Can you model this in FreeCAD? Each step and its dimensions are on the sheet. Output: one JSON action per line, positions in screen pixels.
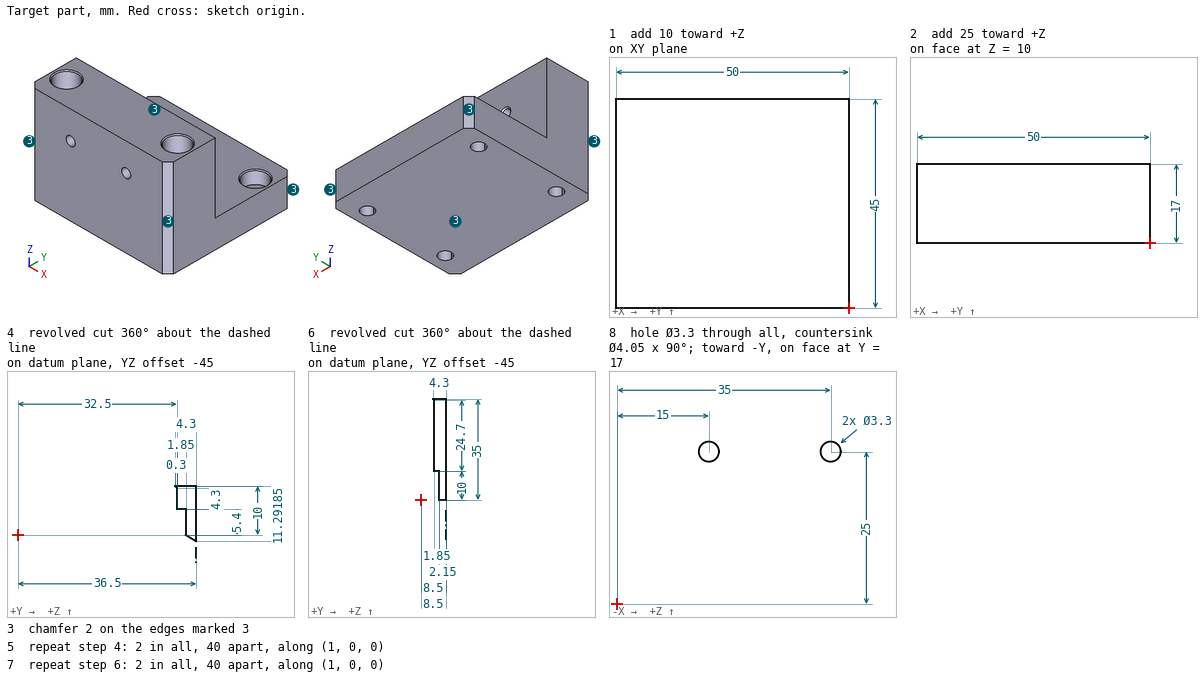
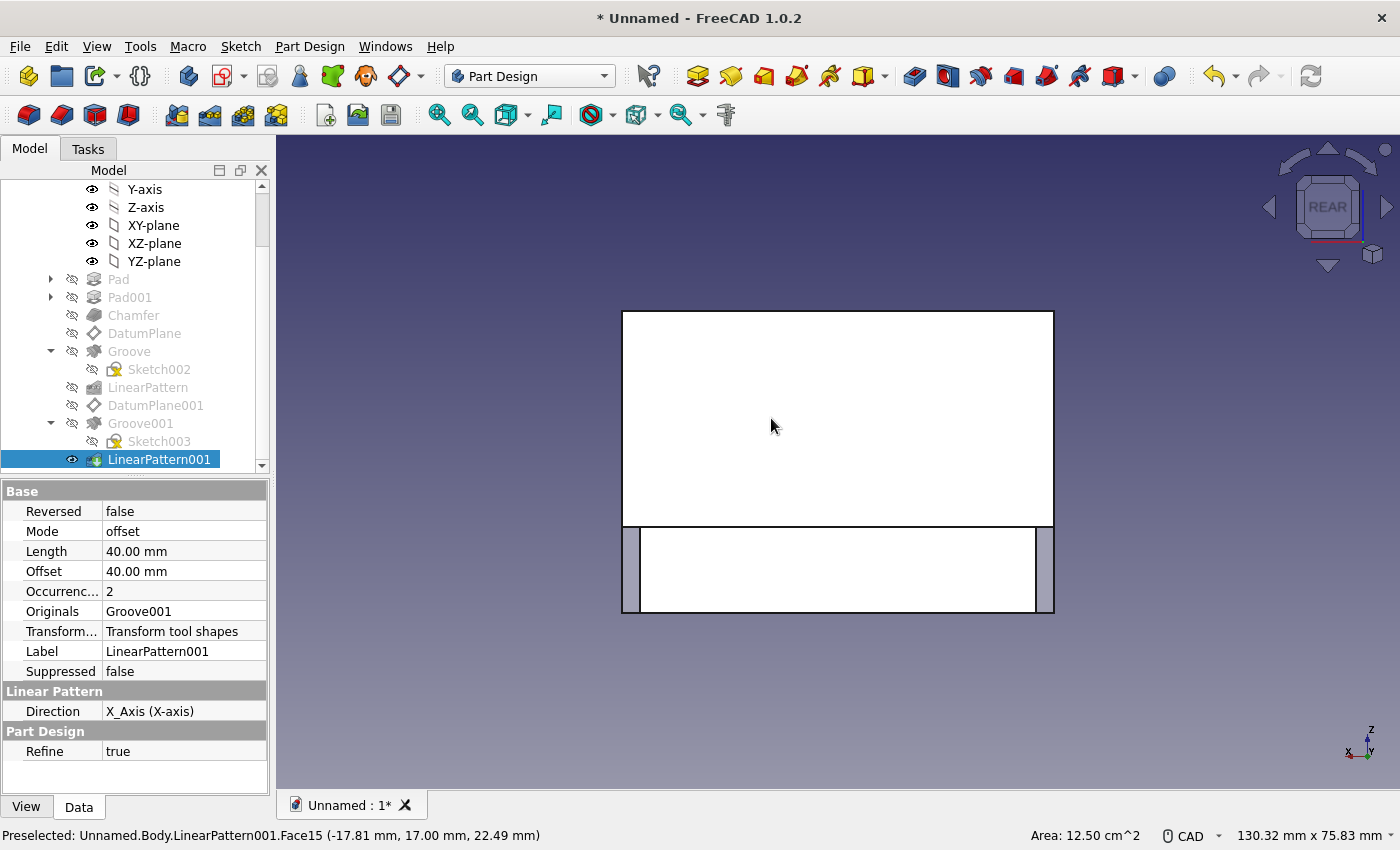
{"action": "left_click", "coordinate": [222, 76]}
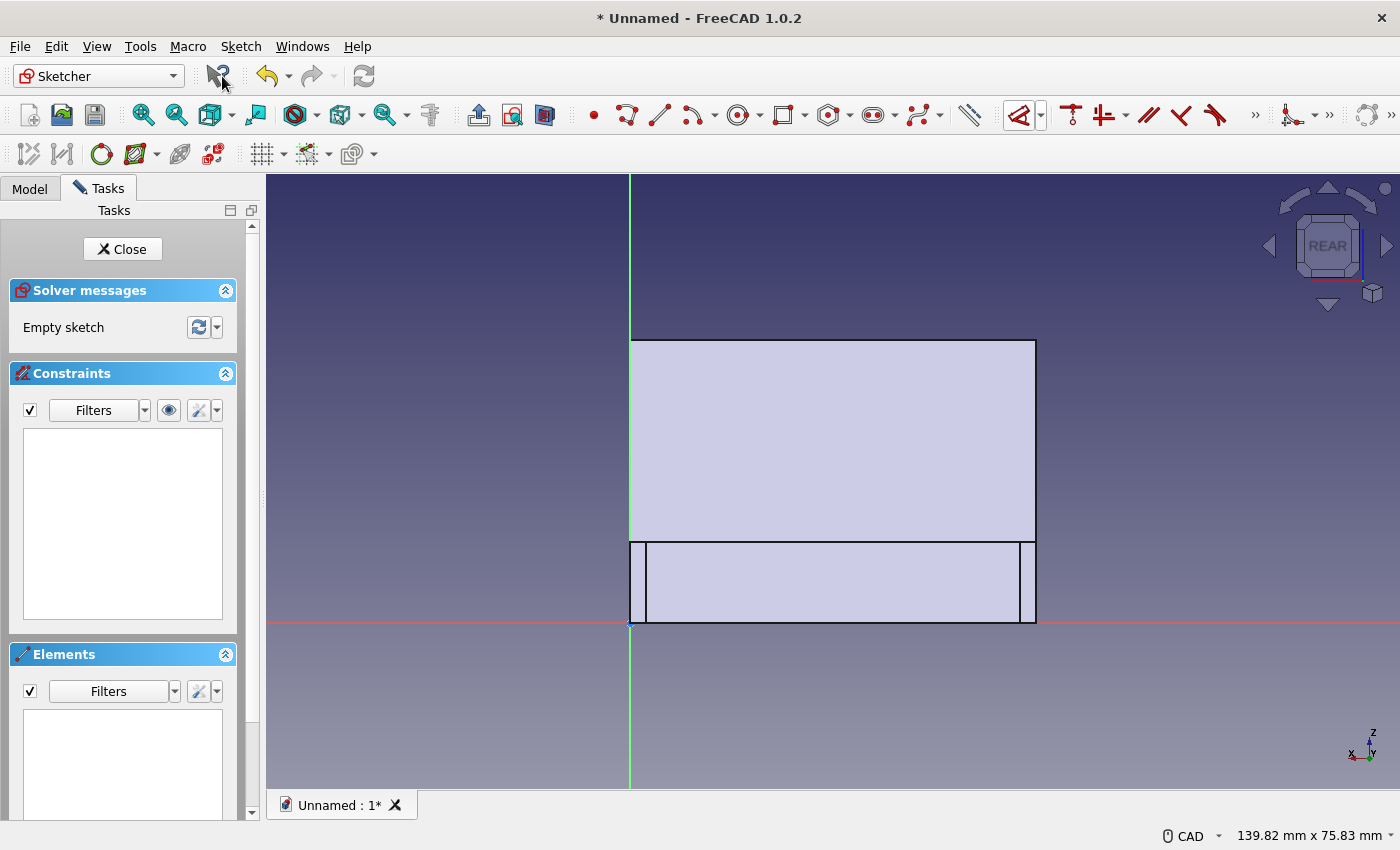
{"action": "scroll", "coordinate": [796, 557], "scroll_direction": "up", "scroll_amount": 3}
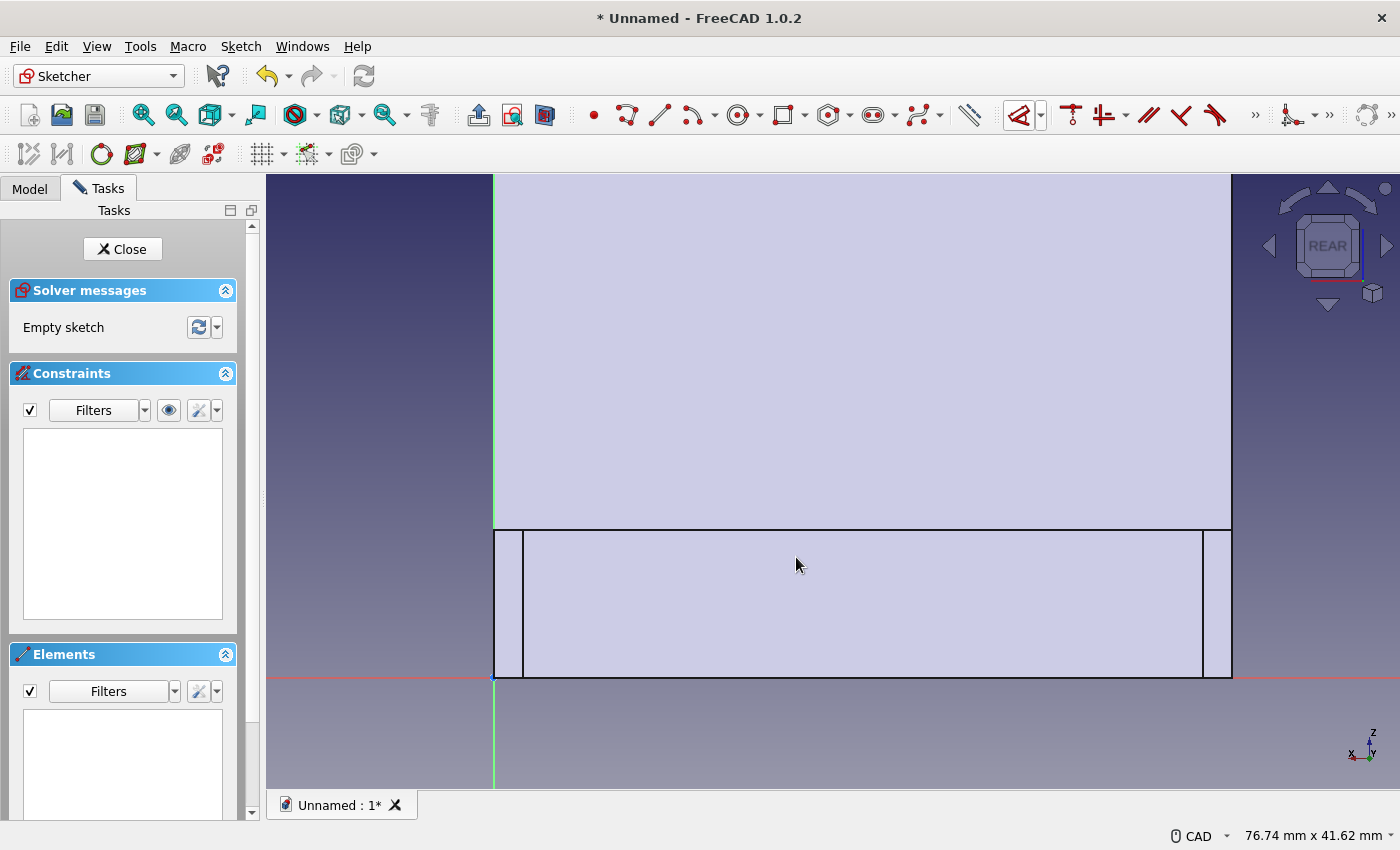
{"action": "left_click", "coordinate": [738, 116]}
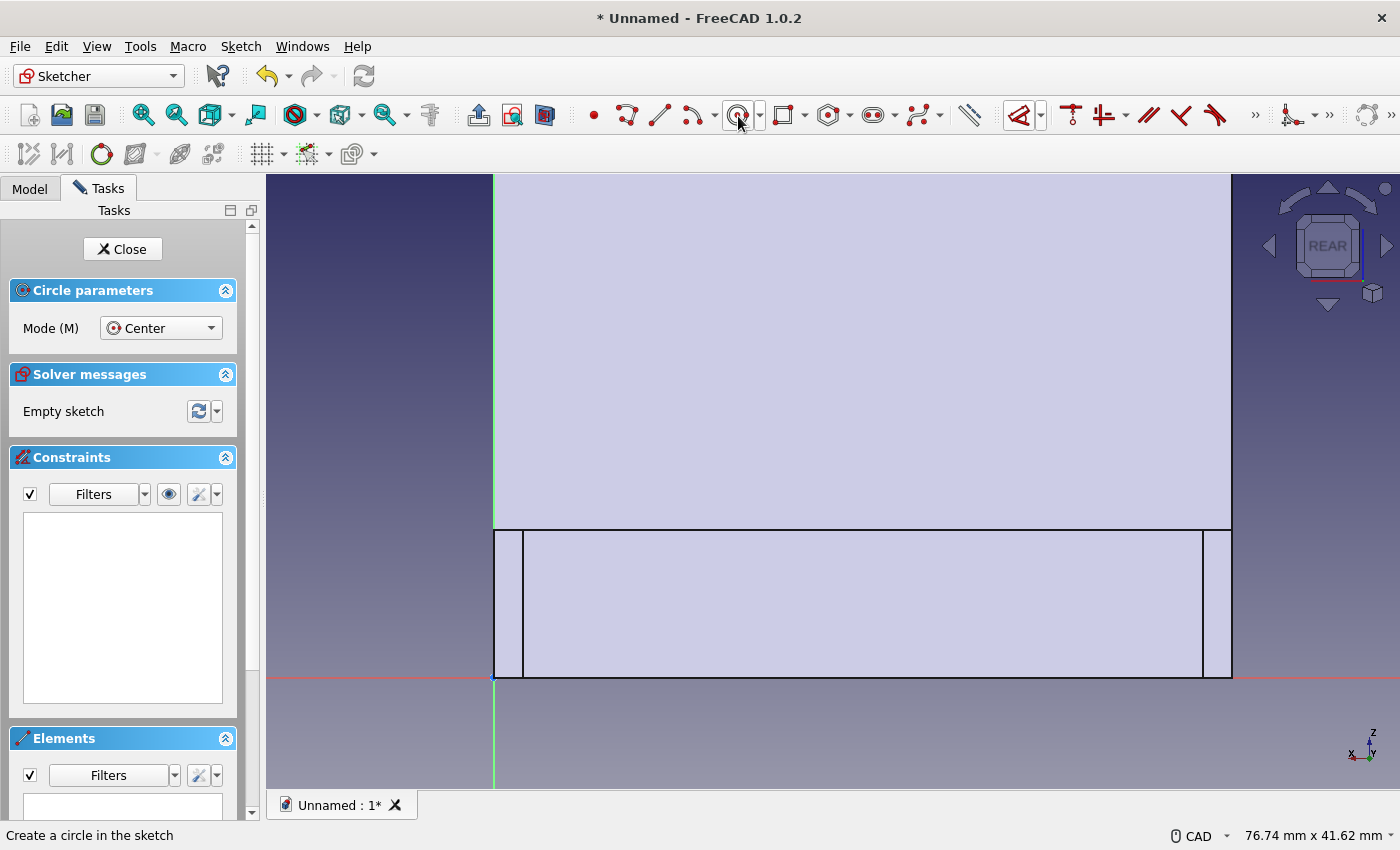
{"action": "left_click", "coordinate": [1011, 308]}
{"action": "left_click", "coordinate": [1028, 291]}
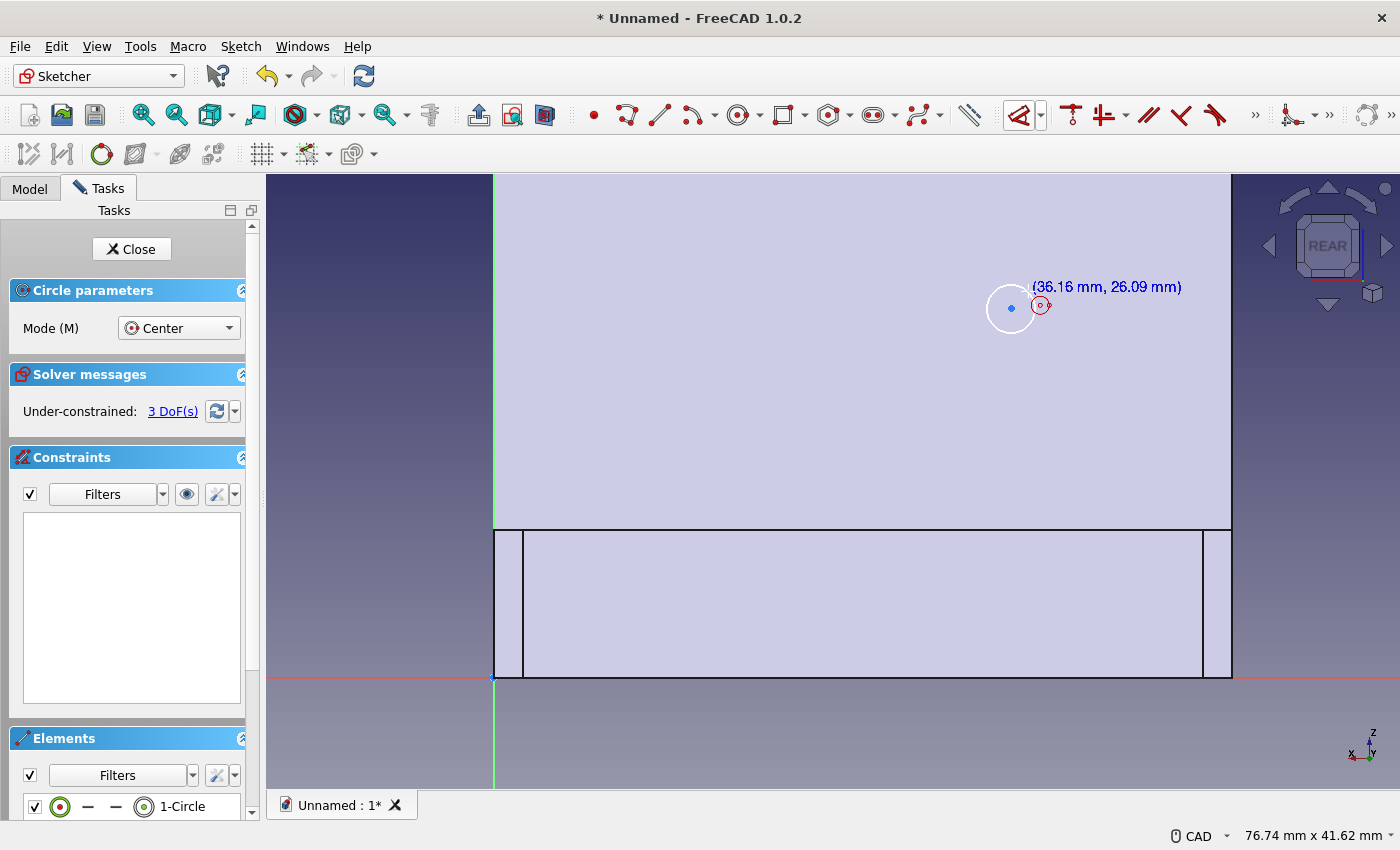
{"action": "left_click", "coordinate": [715, 308]}
{"action": "left_click", "coordinate": [732, 291]}
{"action": "key", "text": "Escape"}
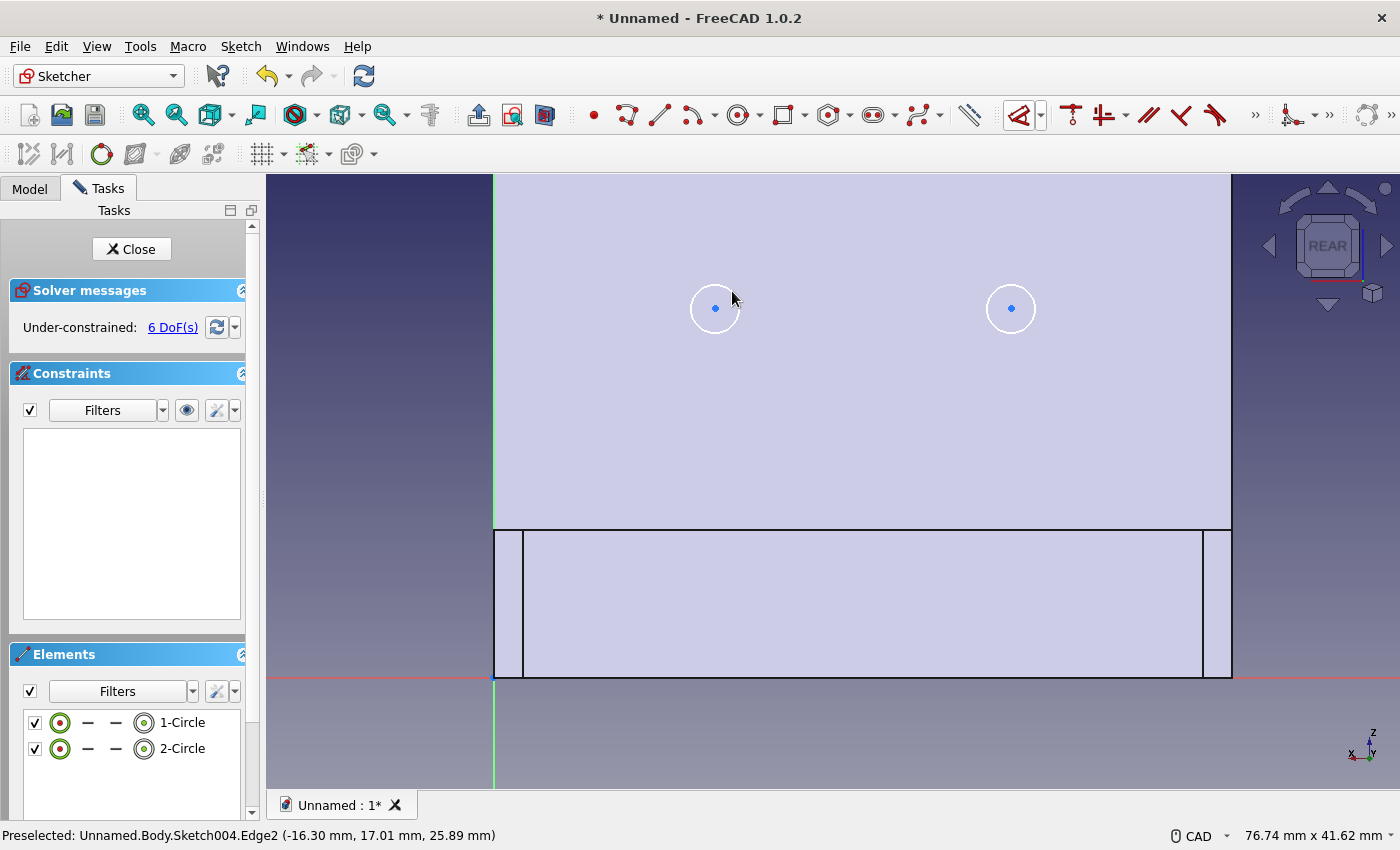
{"action": "left_click", "coordinate": [1028, 292]}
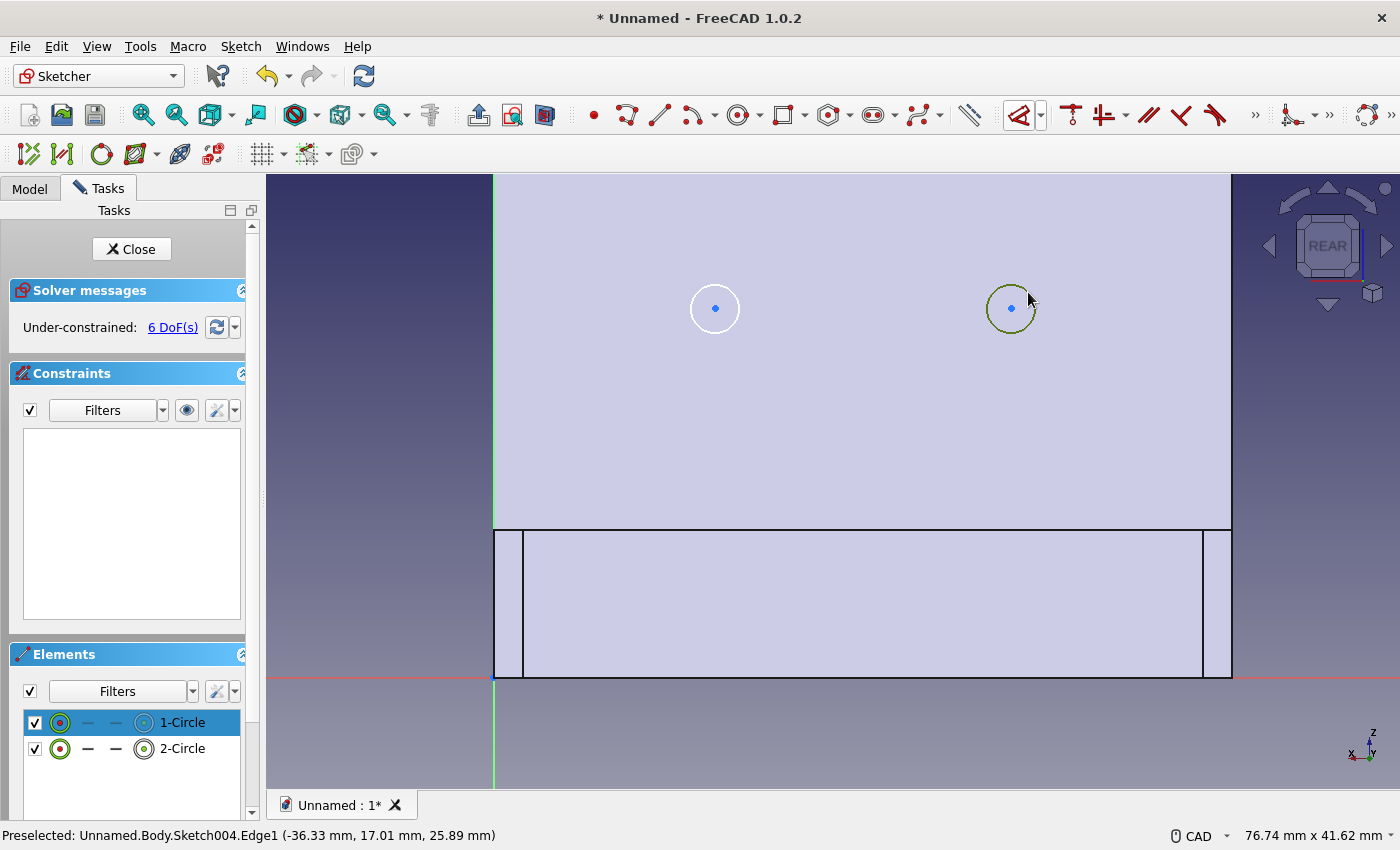
{"action": "left_click", "coordinate": [732, 292]}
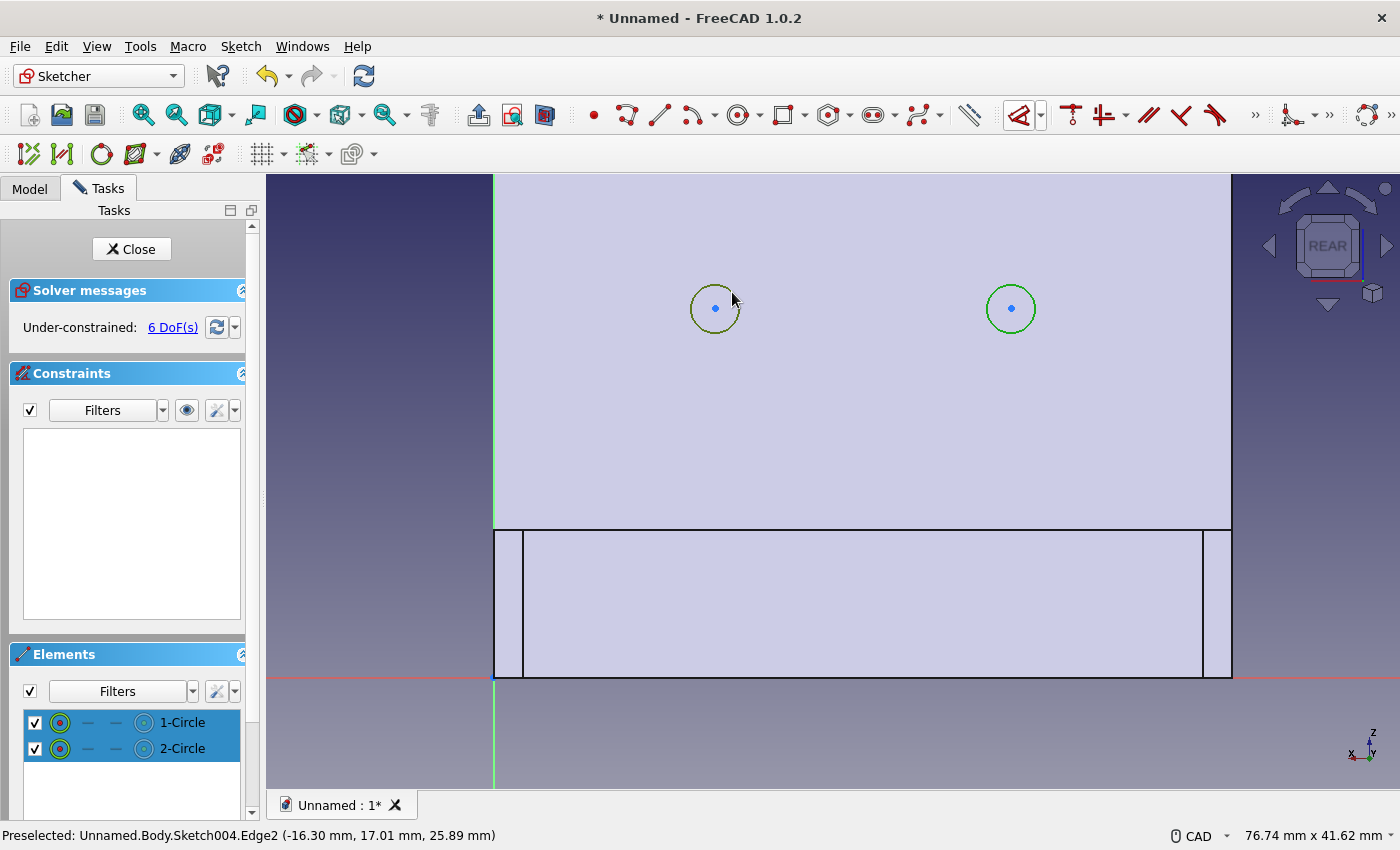
{"action": "key", "text": "e"}